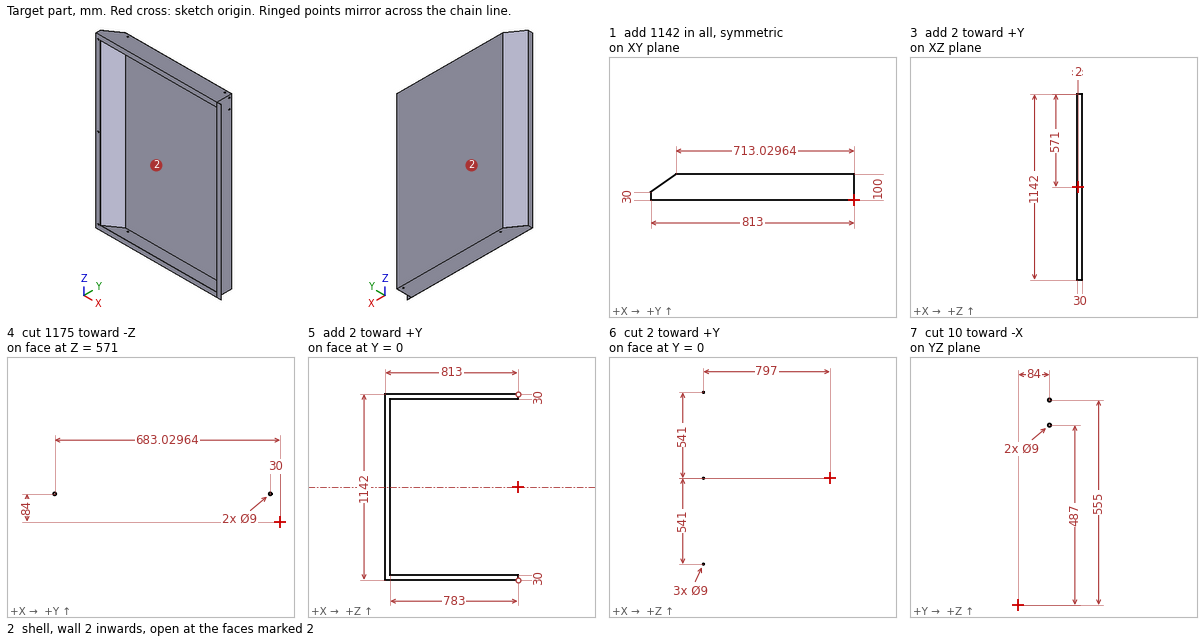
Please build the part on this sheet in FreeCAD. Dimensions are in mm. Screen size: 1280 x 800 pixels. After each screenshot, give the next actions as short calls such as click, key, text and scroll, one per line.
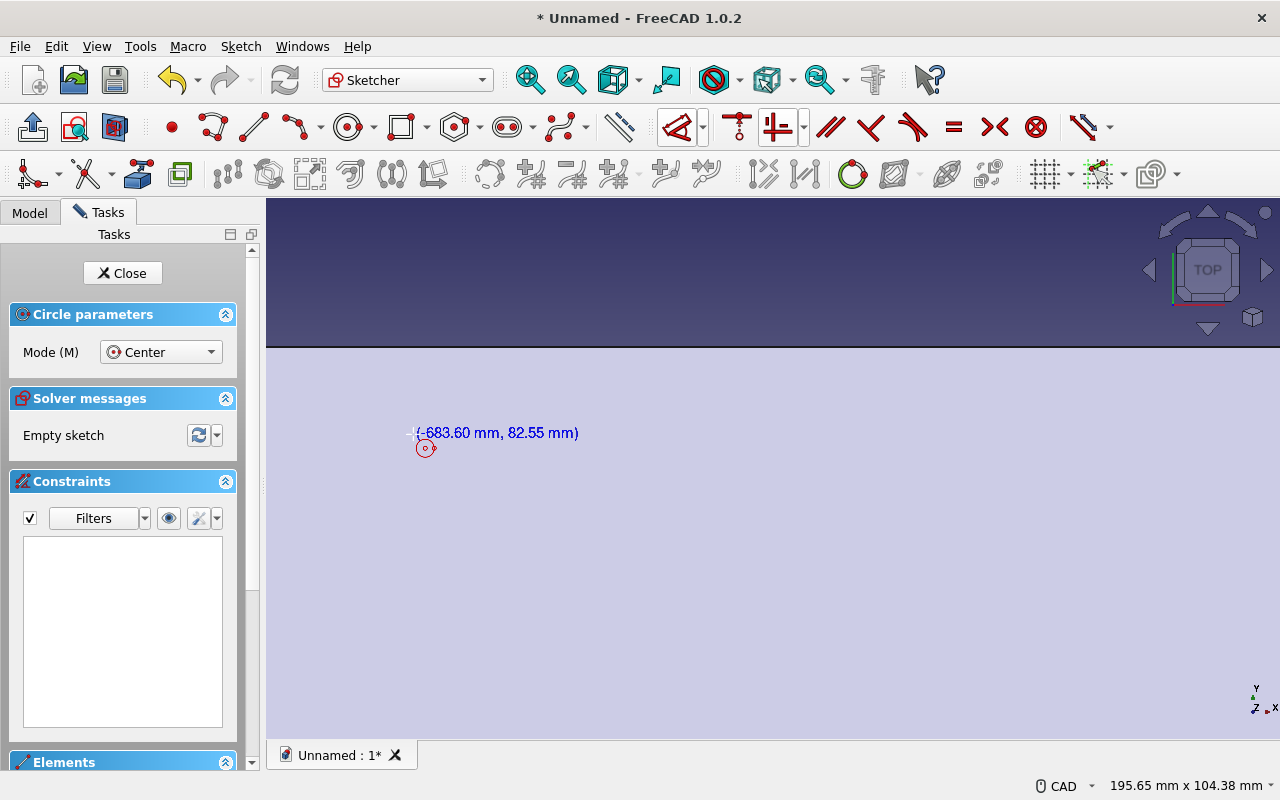
scroll(414, 435, down, 9)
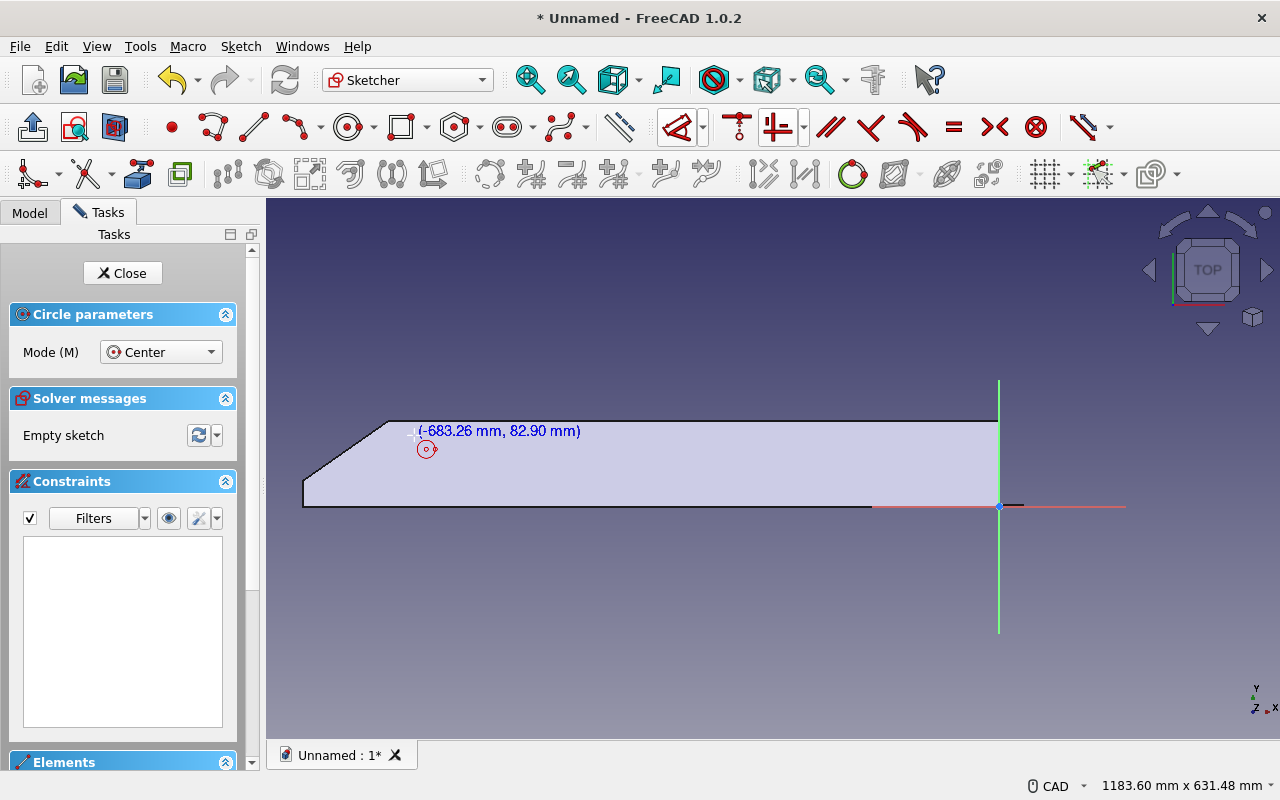
click(414, 435)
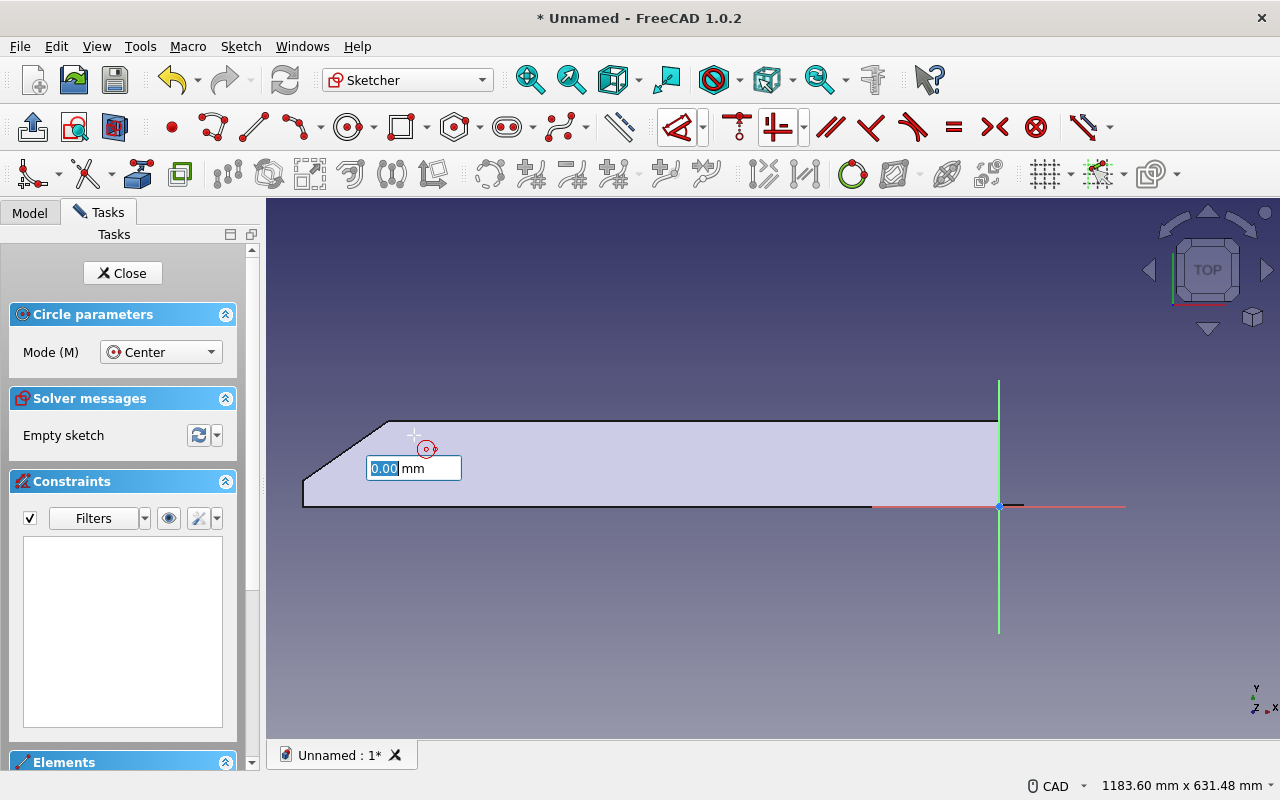
scroll(417, 432, up, 8)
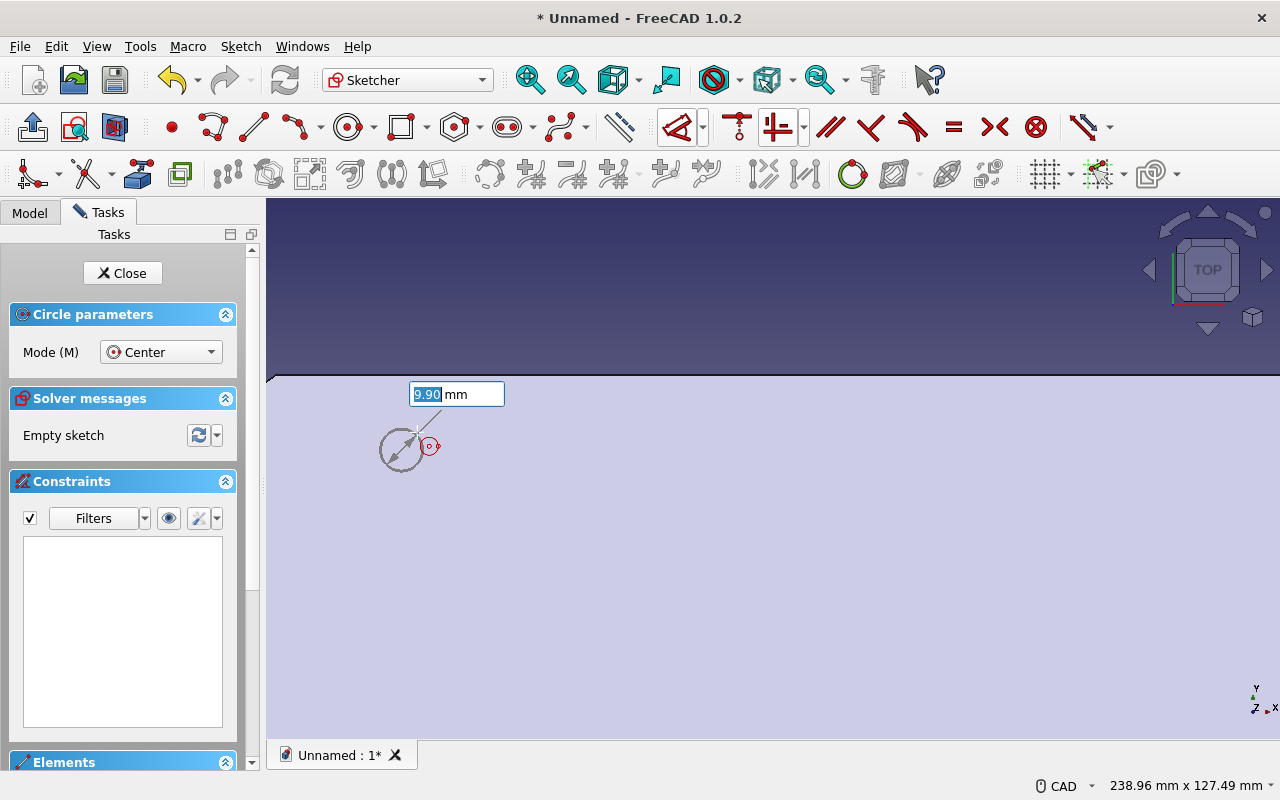
click(417, 430)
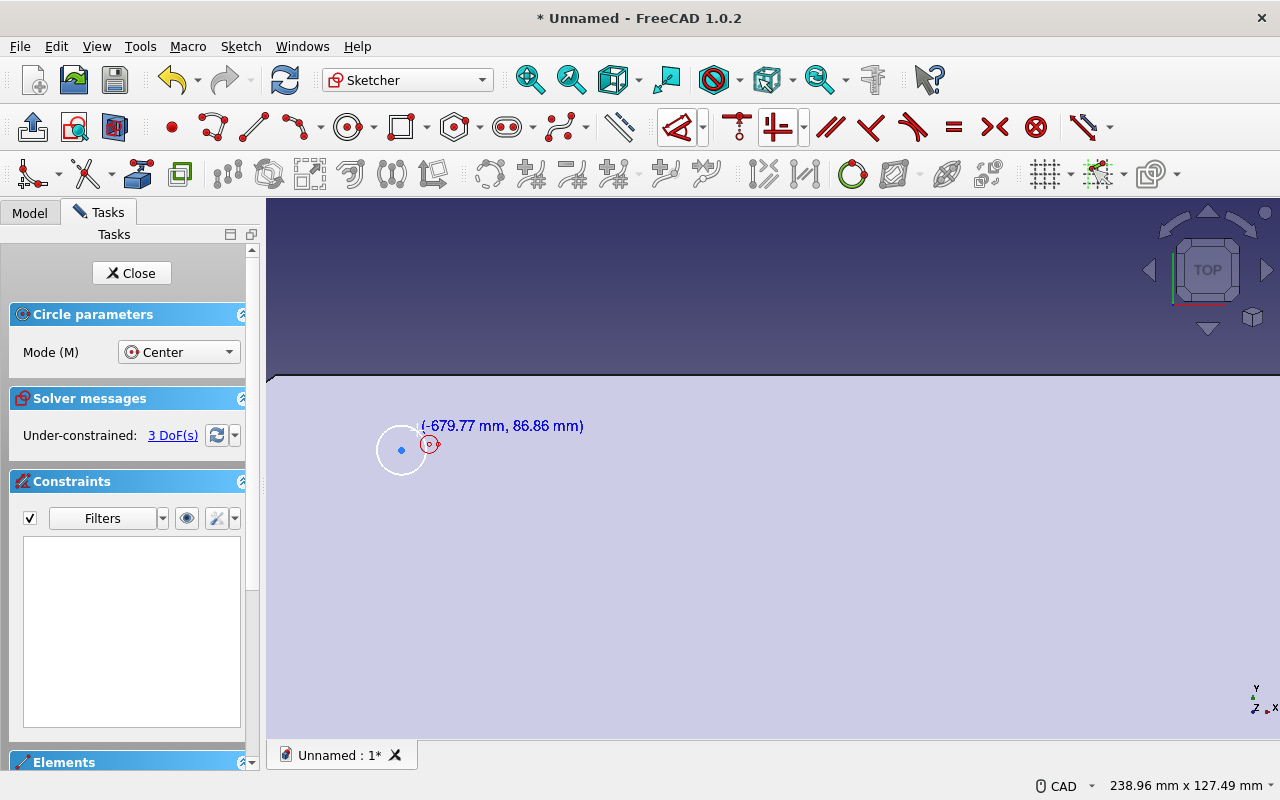
scroll(417, 432, down, 8)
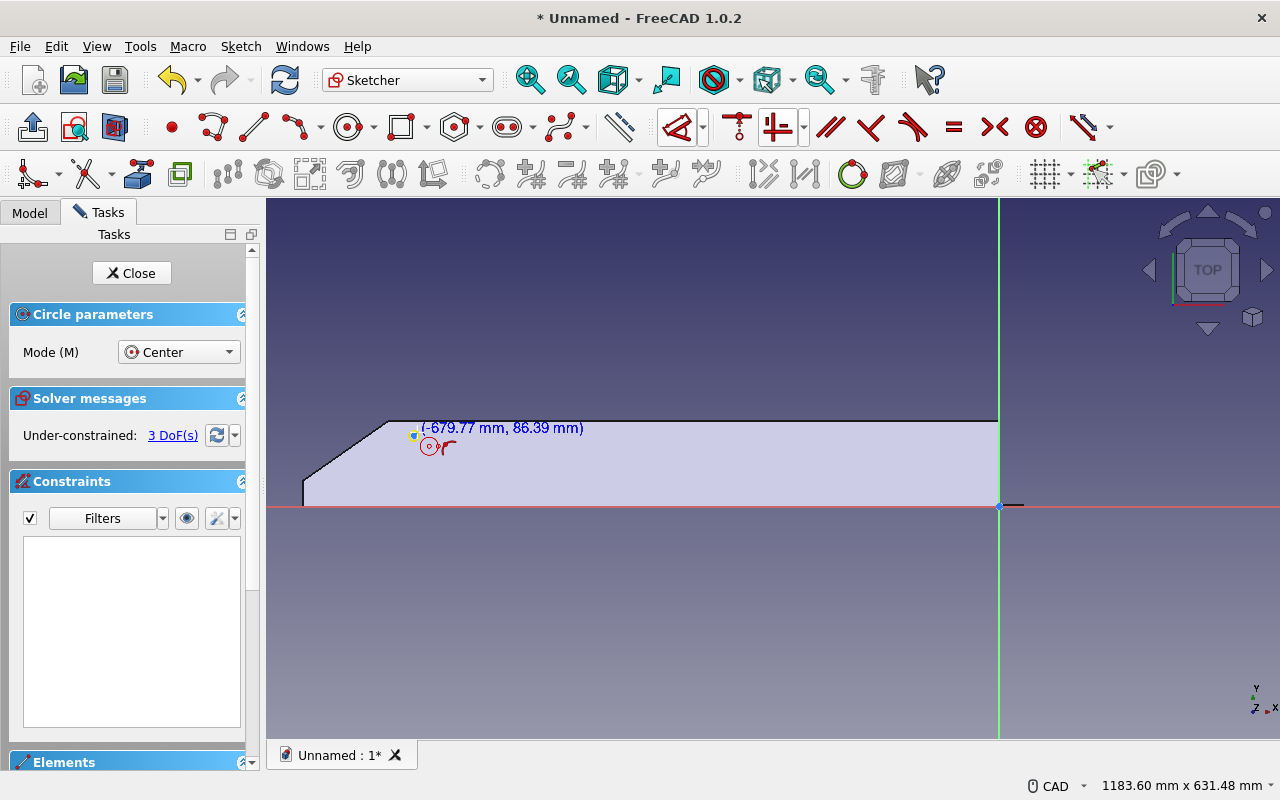
scroll(974, 435, up, 9)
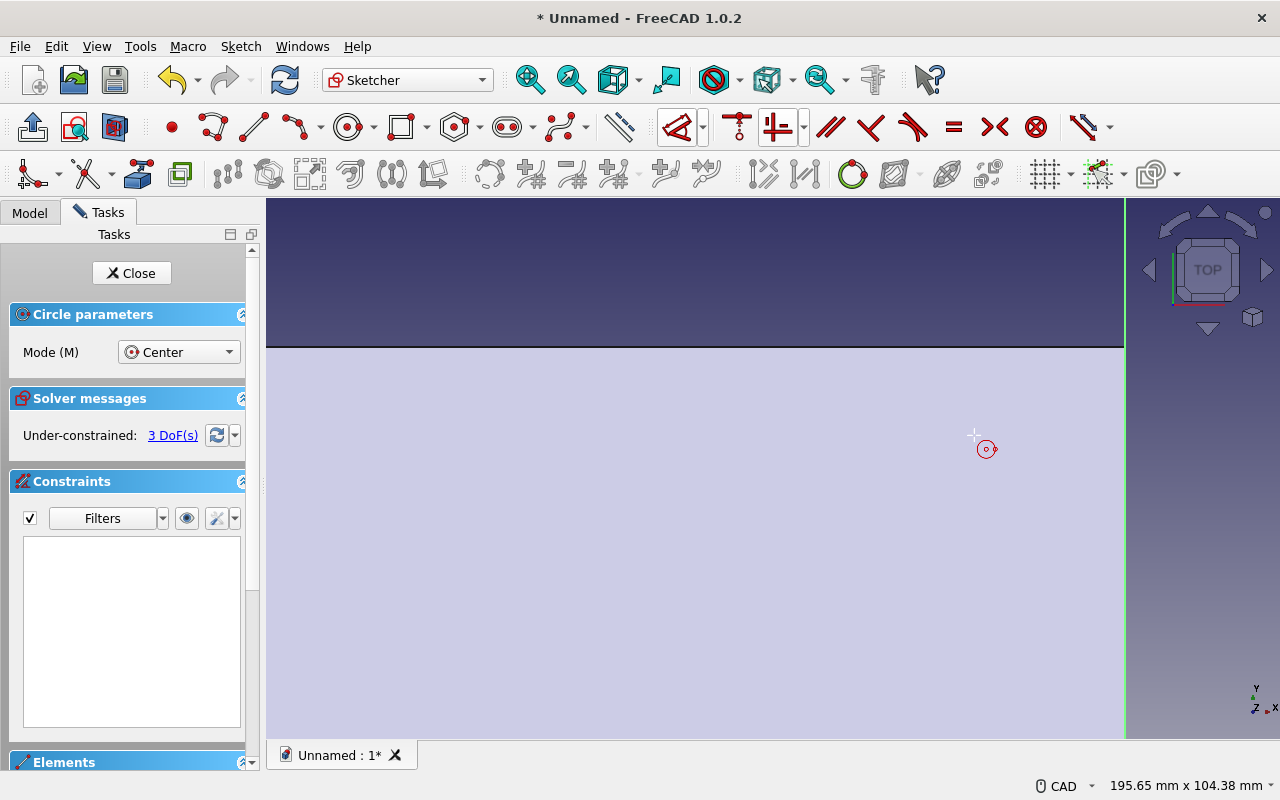
scroll(974, 435, down, 9)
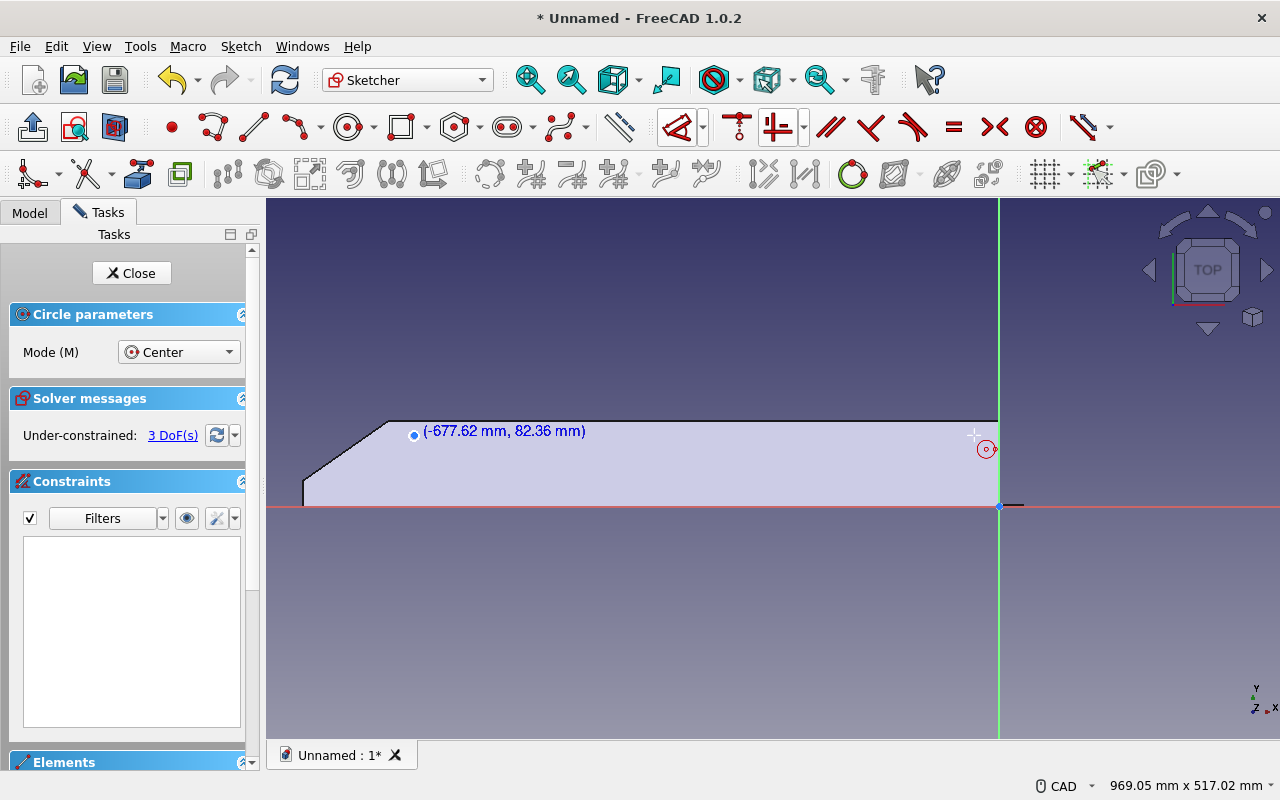
click(974, 435)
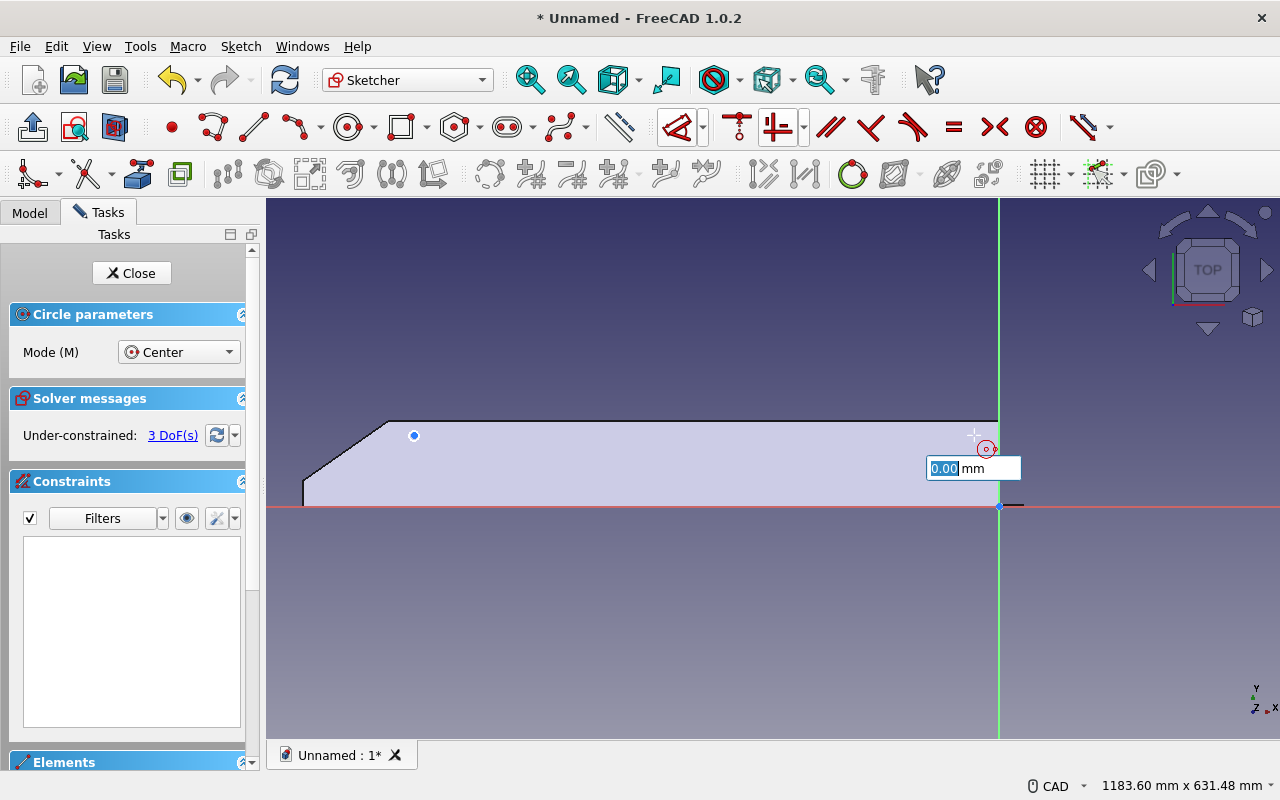
scroll(977, 432, up, 8)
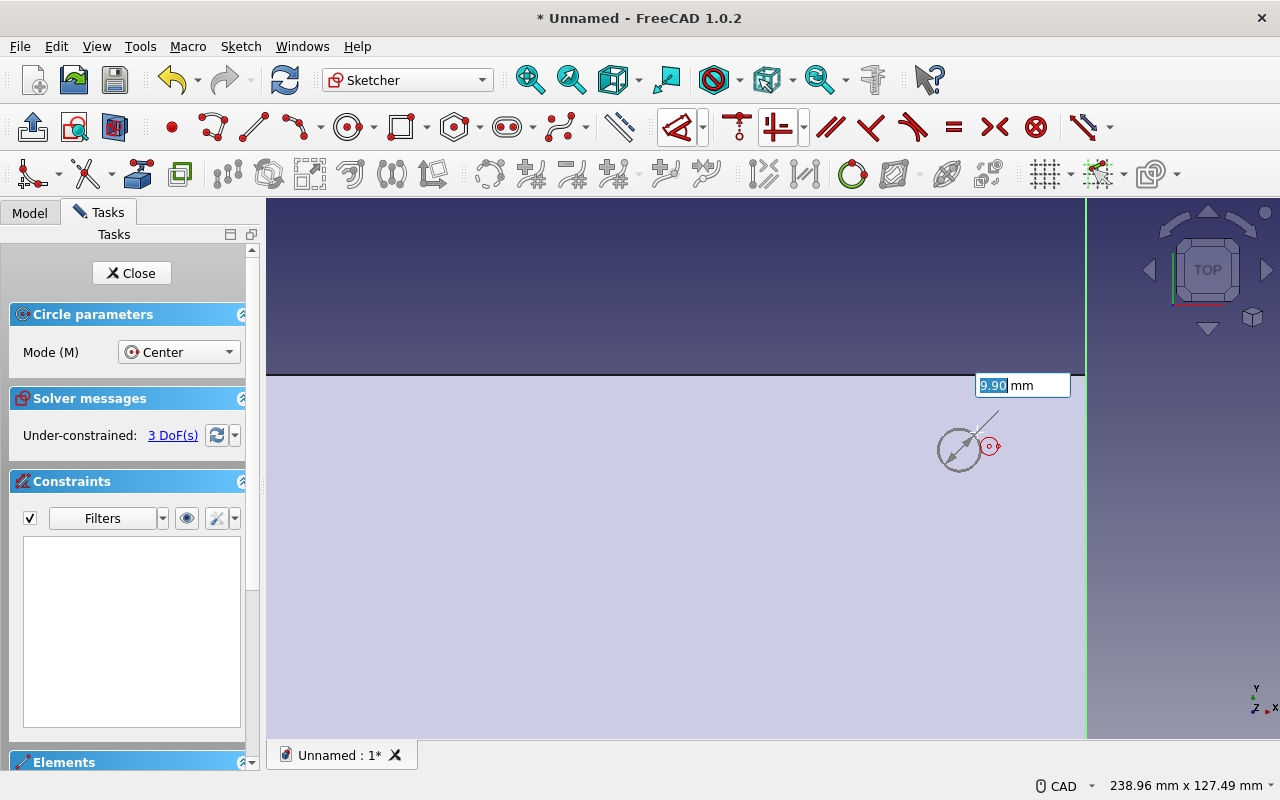
click(972, 430)
key(Escape)